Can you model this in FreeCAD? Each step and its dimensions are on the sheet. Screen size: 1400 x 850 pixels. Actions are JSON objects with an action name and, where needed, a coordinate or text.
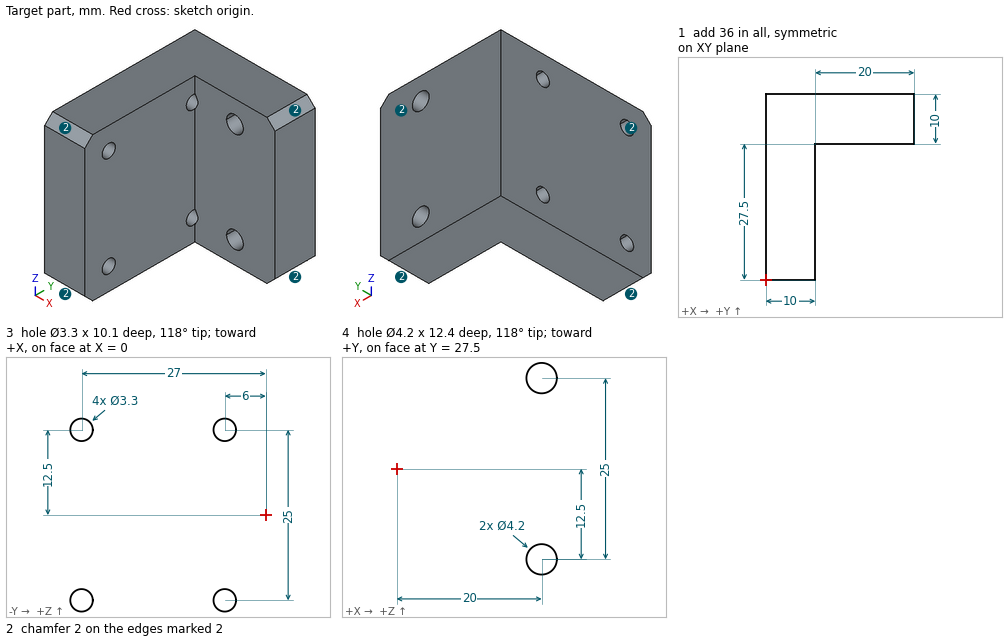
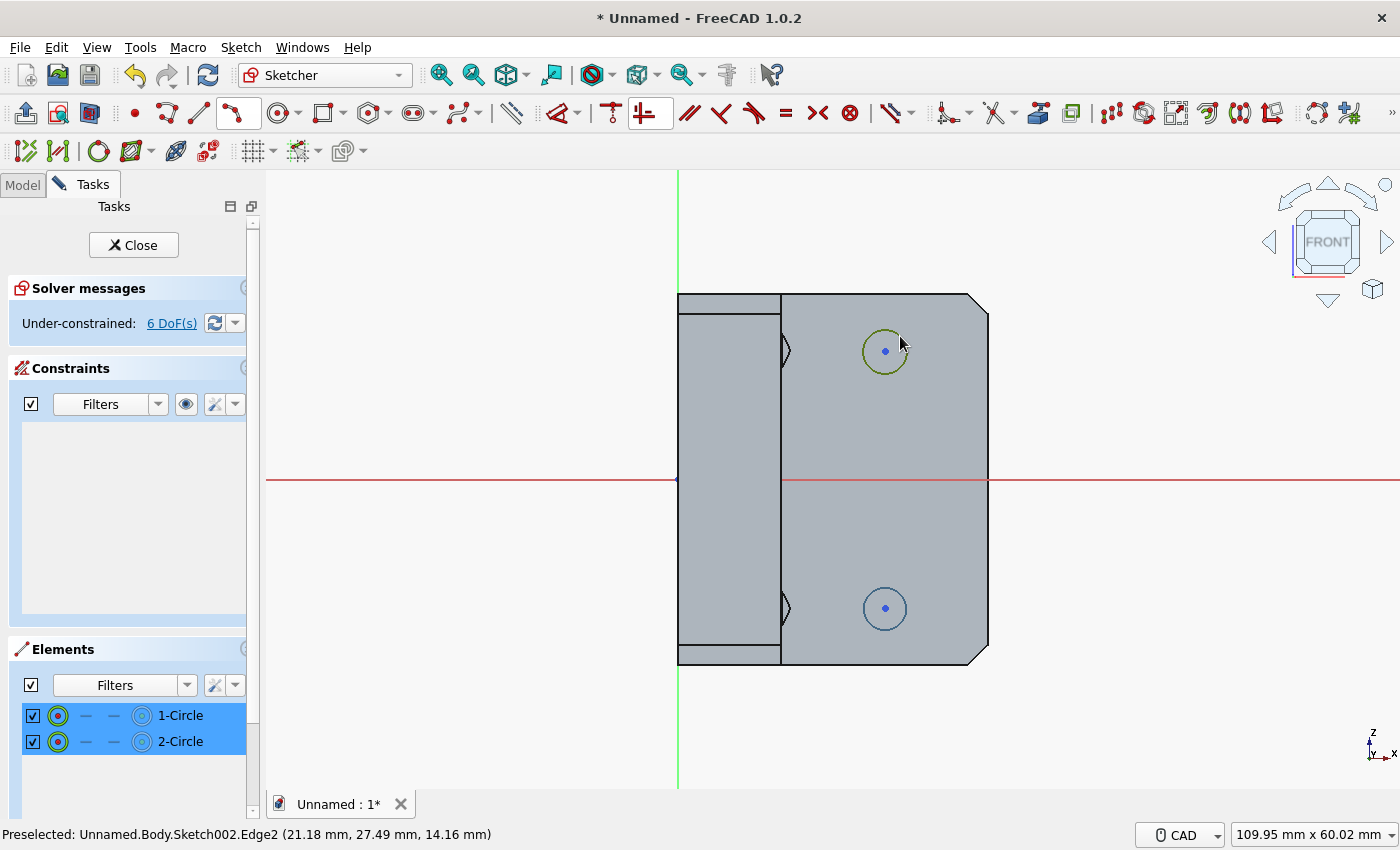
{"action": "left_click", "coordinate": [786, 114]}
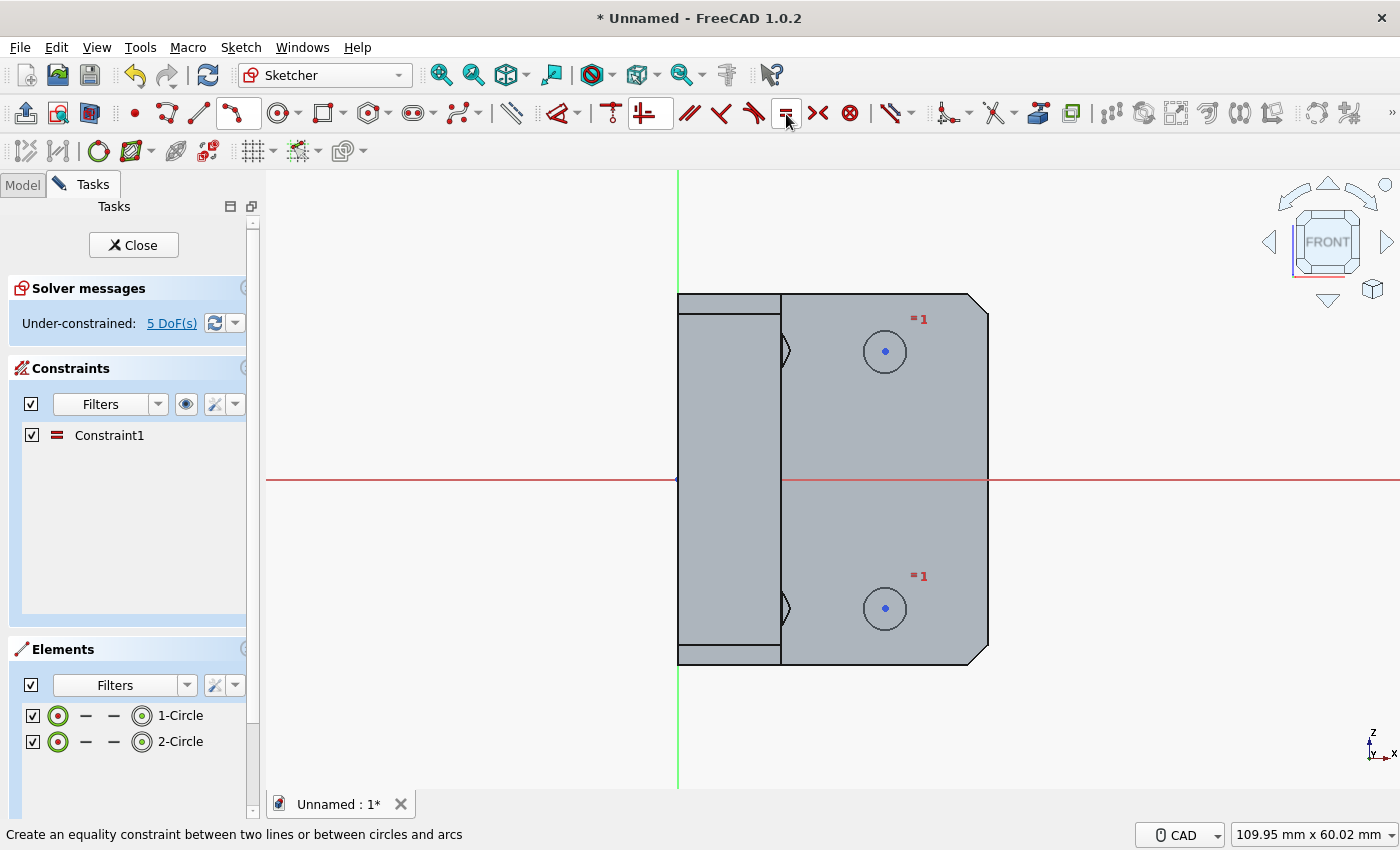
{"action": "left_click", "coordinate": [885, 609]}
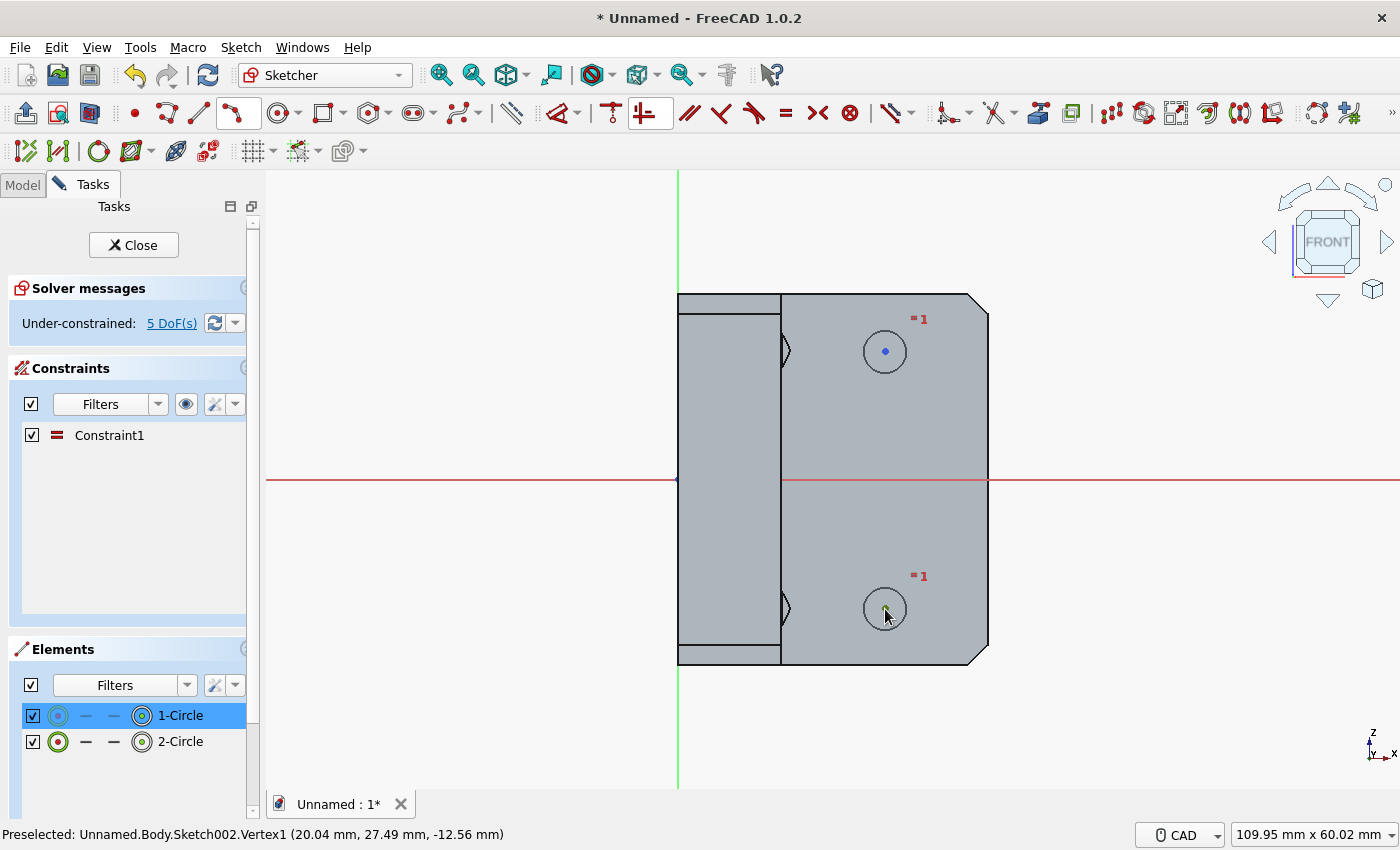
{"action": "left_click", "coordinate": [885, 352]}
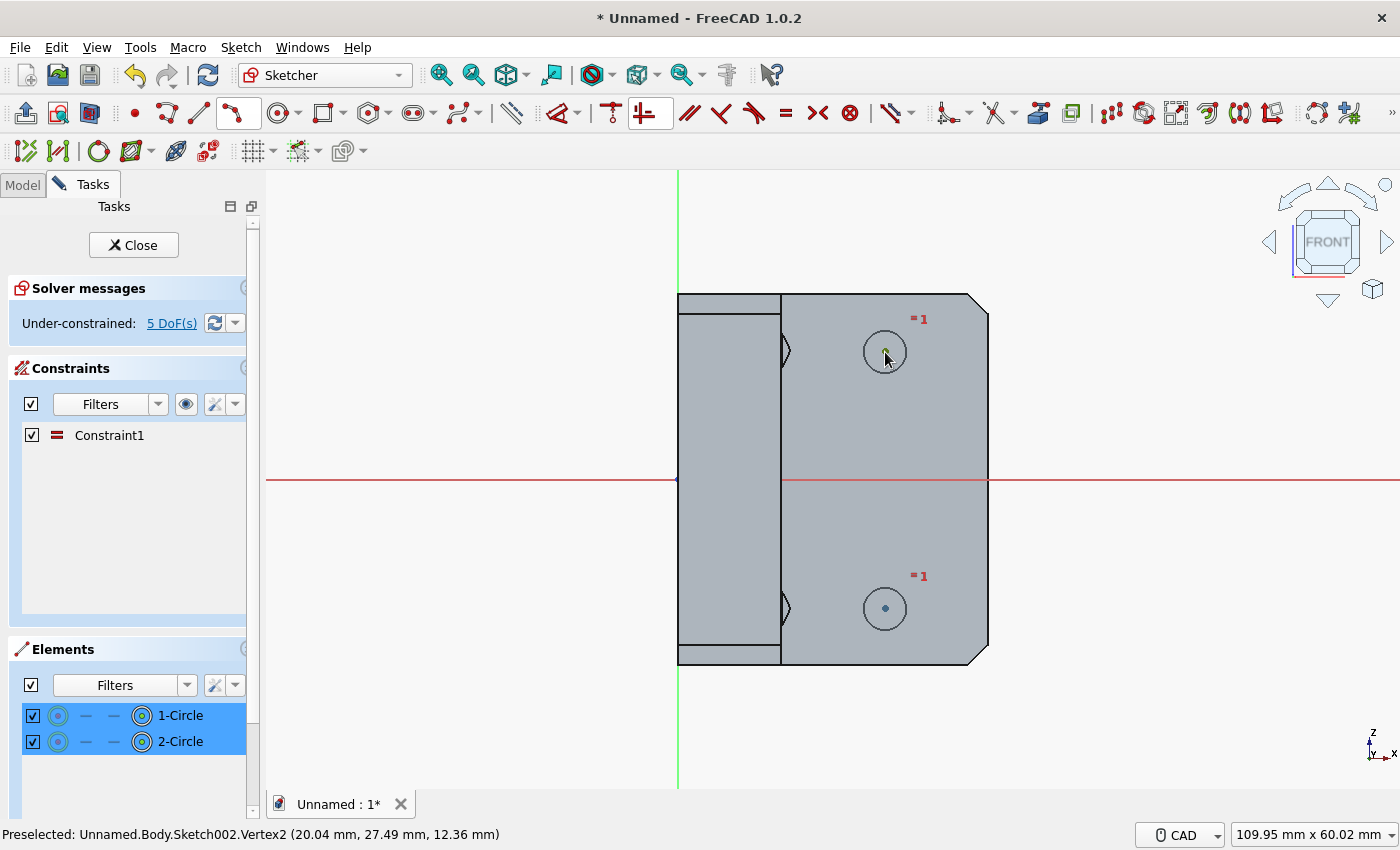
{"action": "key", "text": "v"}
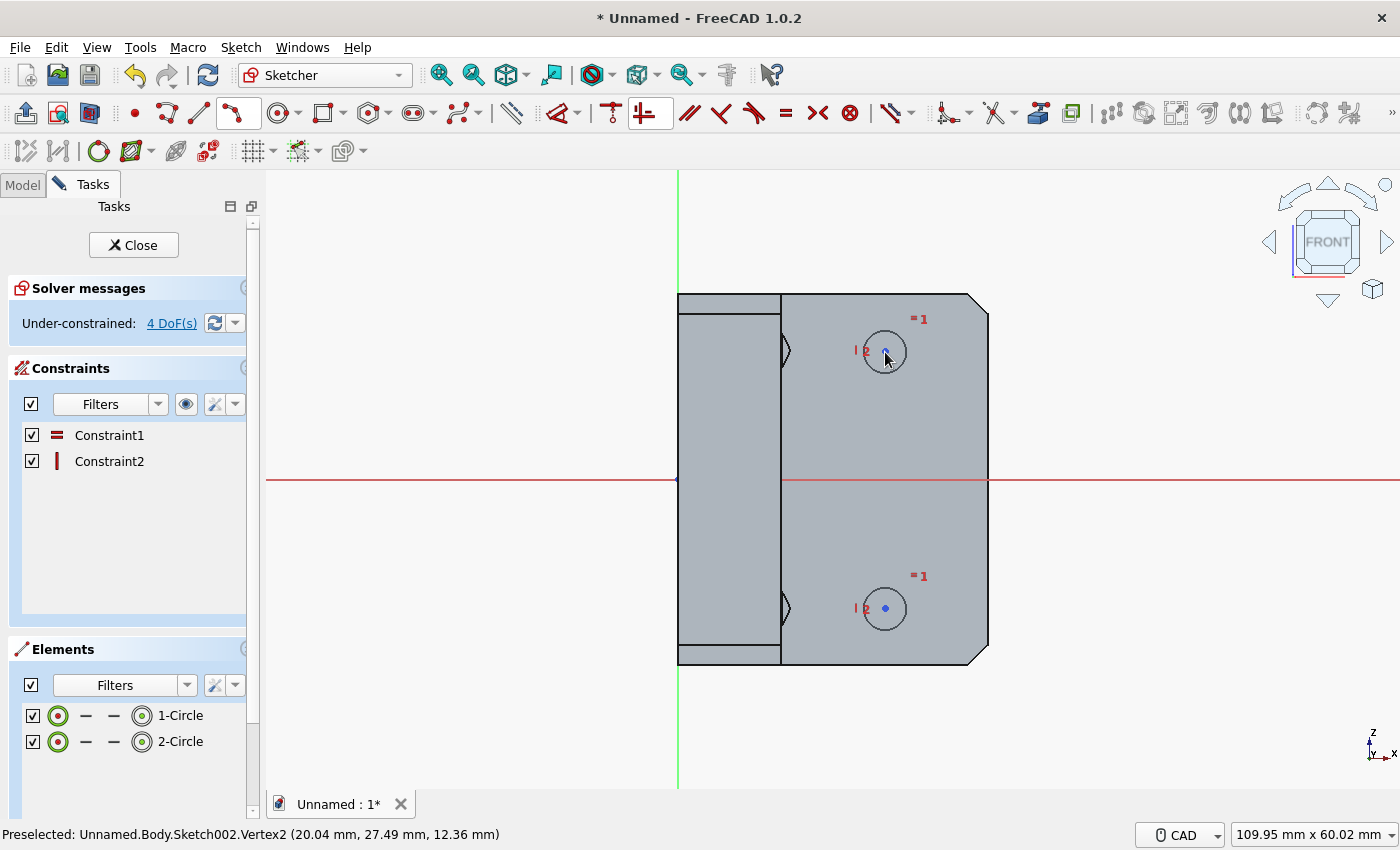
{"action": "left_click", "coordinate": [558, 114]}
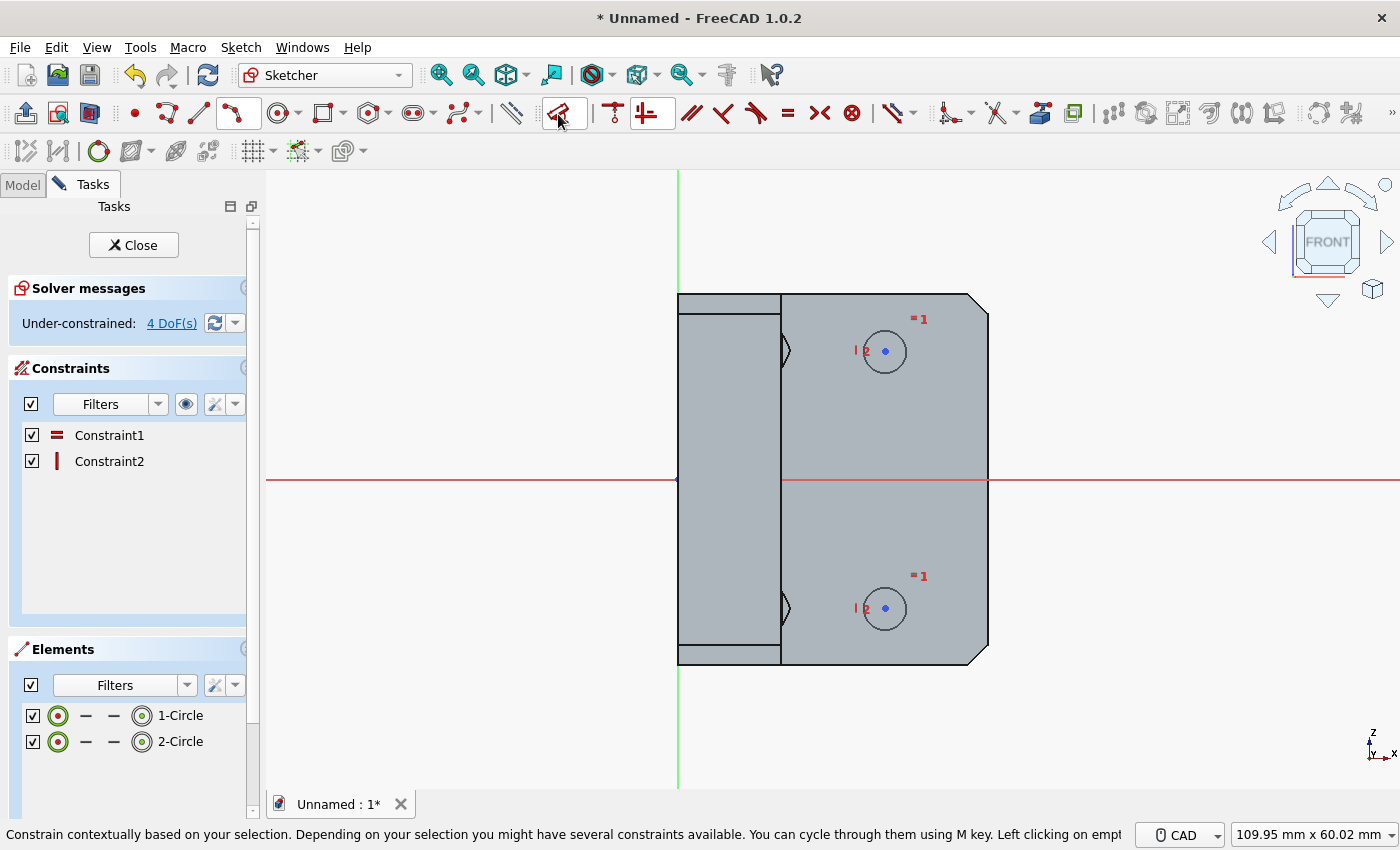
{"action": "left_click", "coordinate": [900, 594]}
{"action": "left_click", "coordinate": [923, 571]}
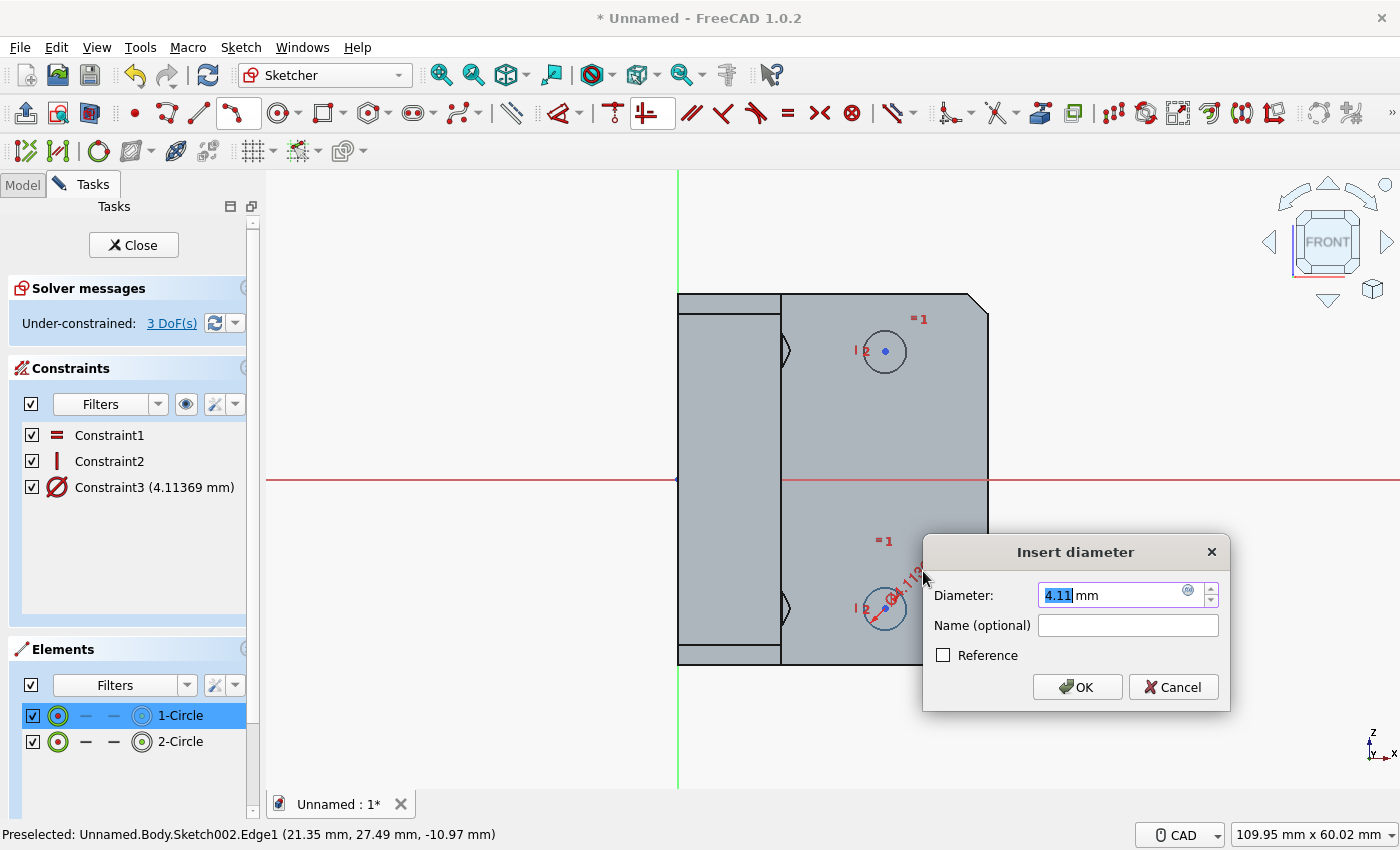
{"action": "type", "text": "4.2"}
{"action": "key", "text": "Return"}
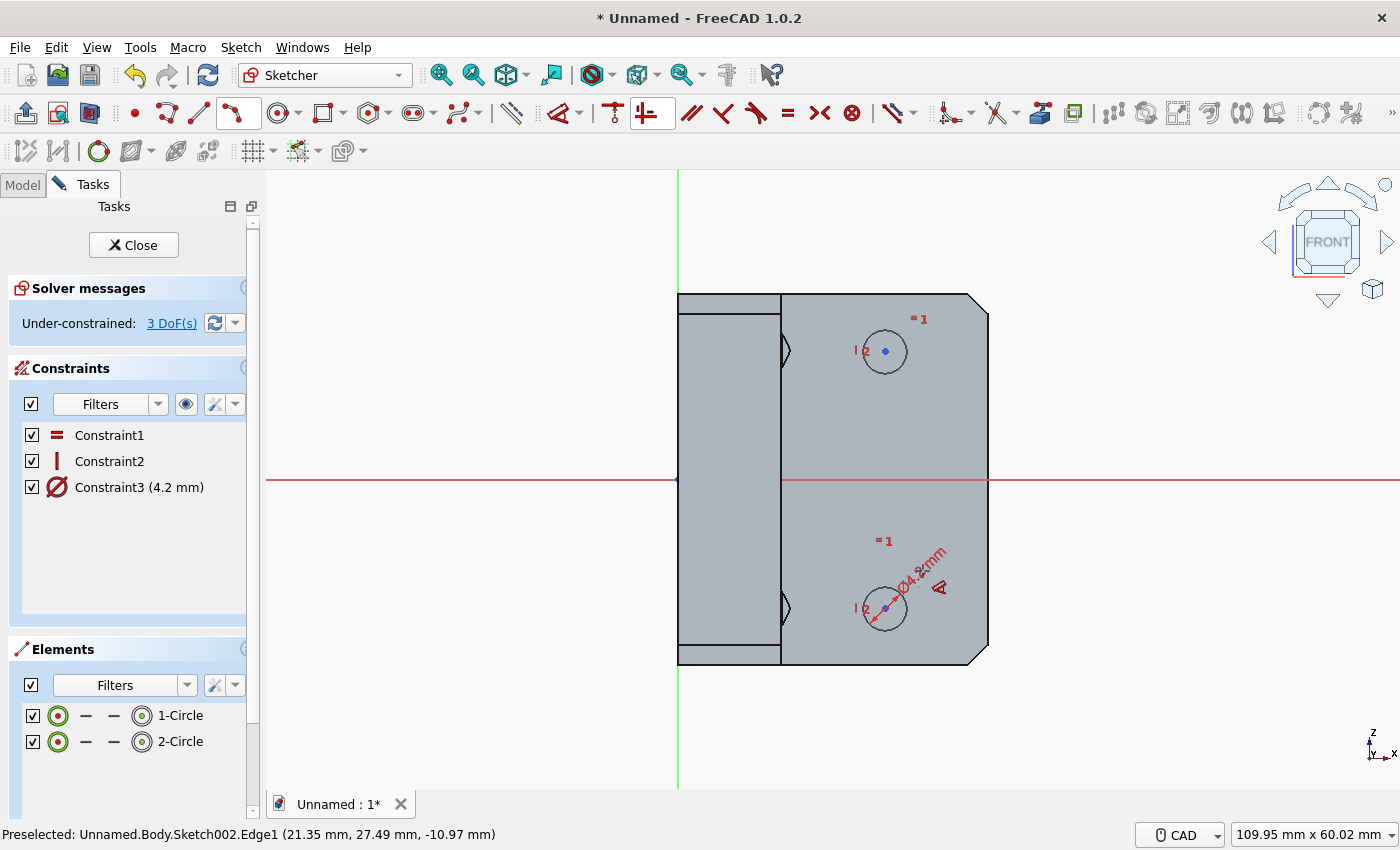
{"action": "left_click", "coordinate": [885, 609]}
{"action": "left_click", "coordinate": [782, 643]}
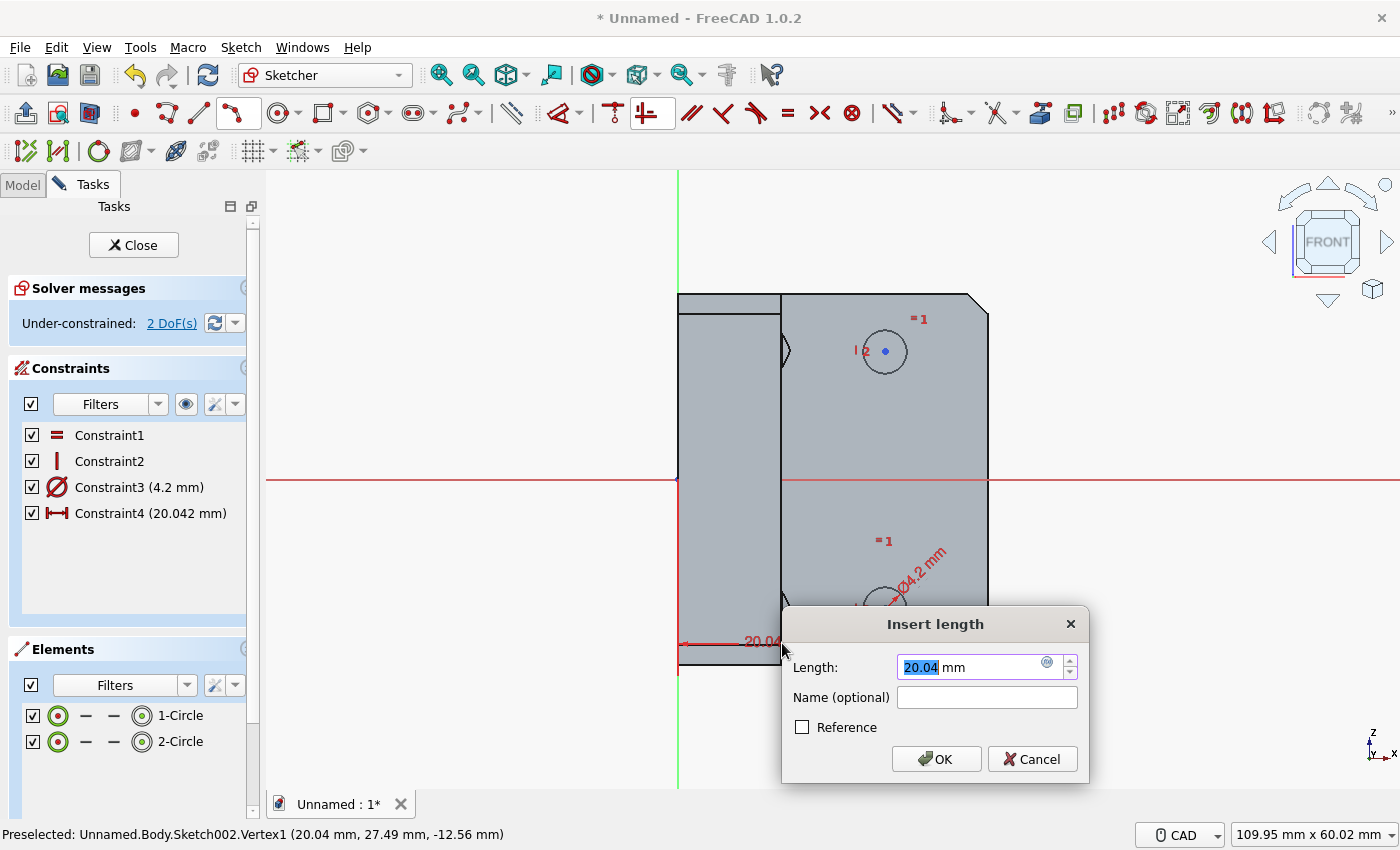
{"action": "type", "text": "20"}
{"action": "key", "text": "Return"}